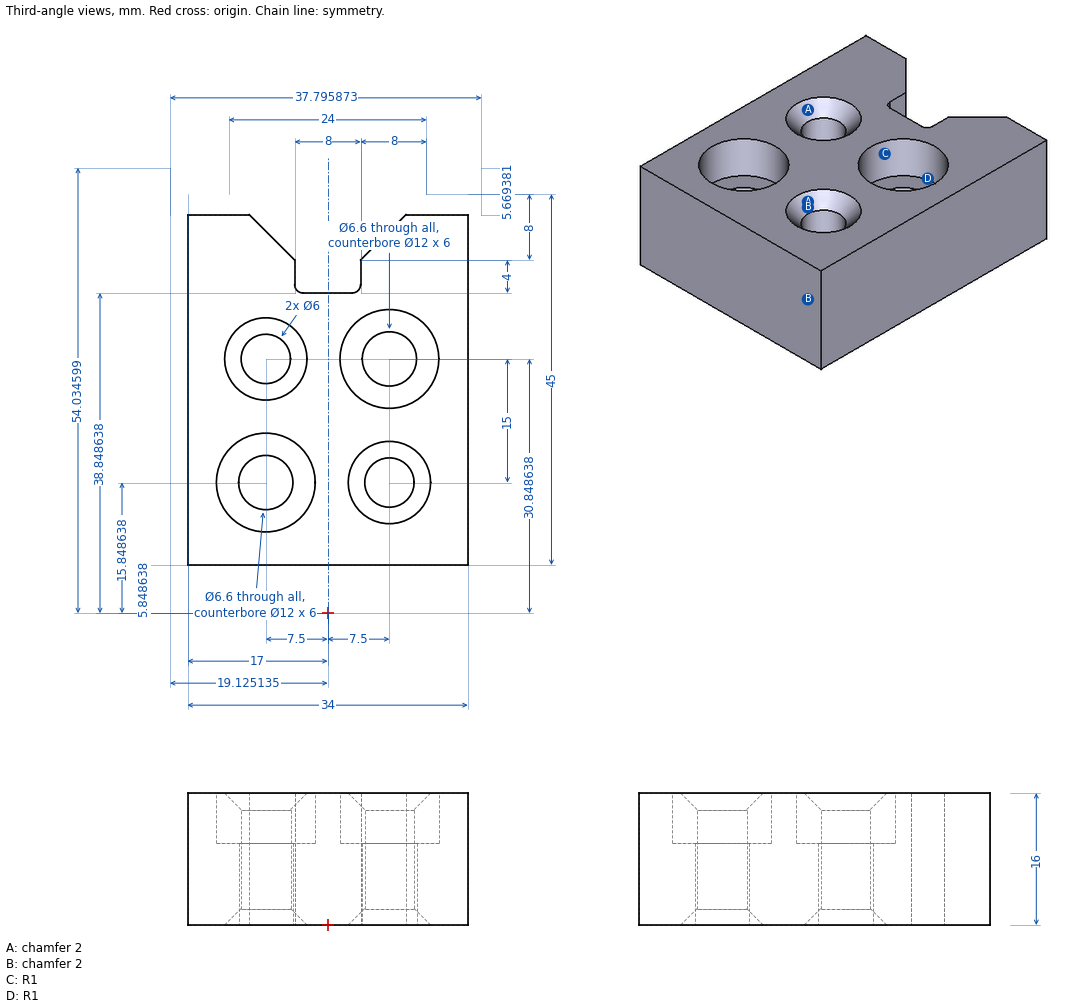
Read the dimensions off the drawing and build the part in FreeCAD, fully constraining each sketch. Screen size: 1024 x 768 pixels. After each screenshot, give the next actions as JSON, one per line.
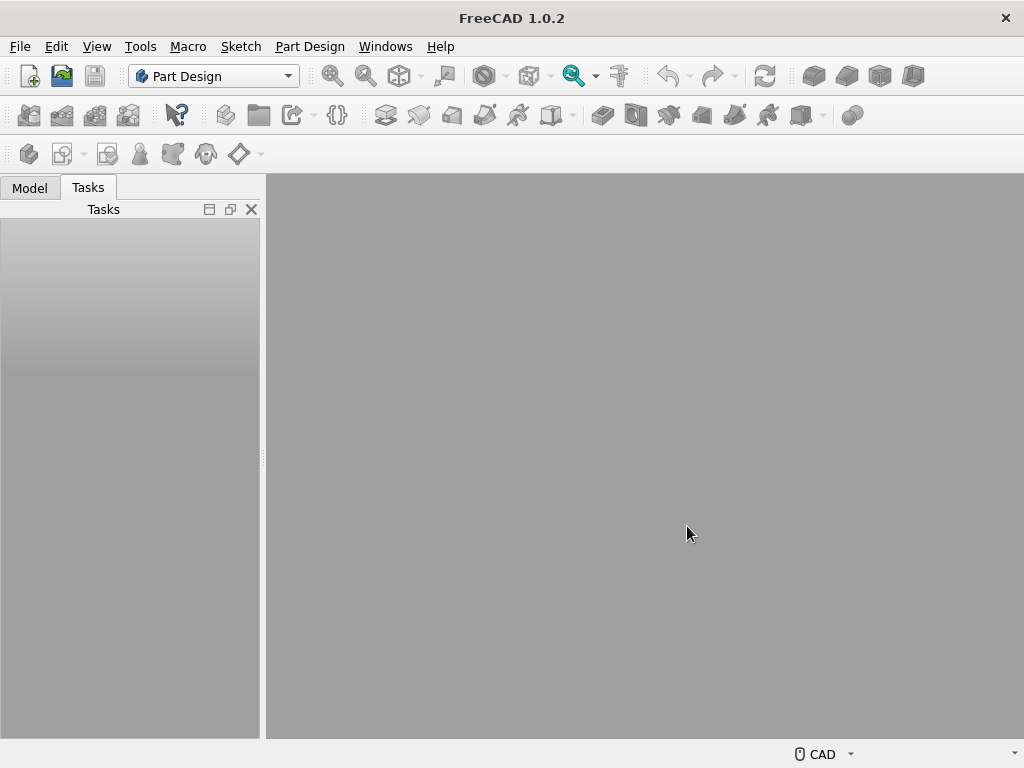
{"action": "left_click", "coordinate": [29, 76]}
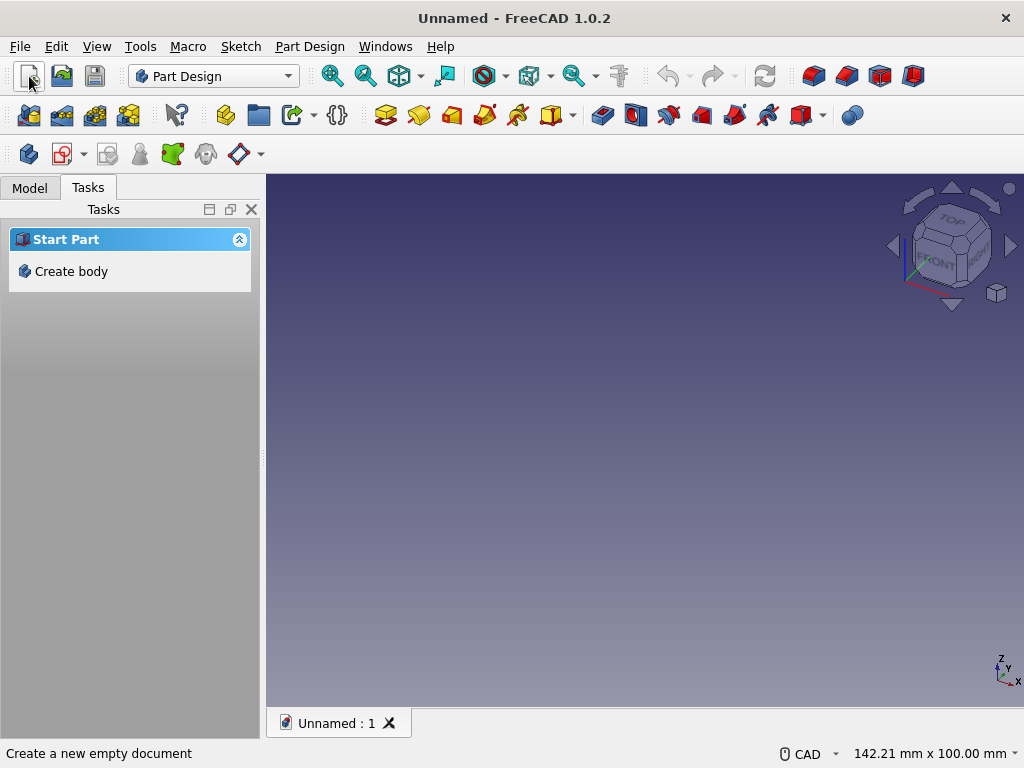
{"action": "left_click", "coordinate": [62, 154]}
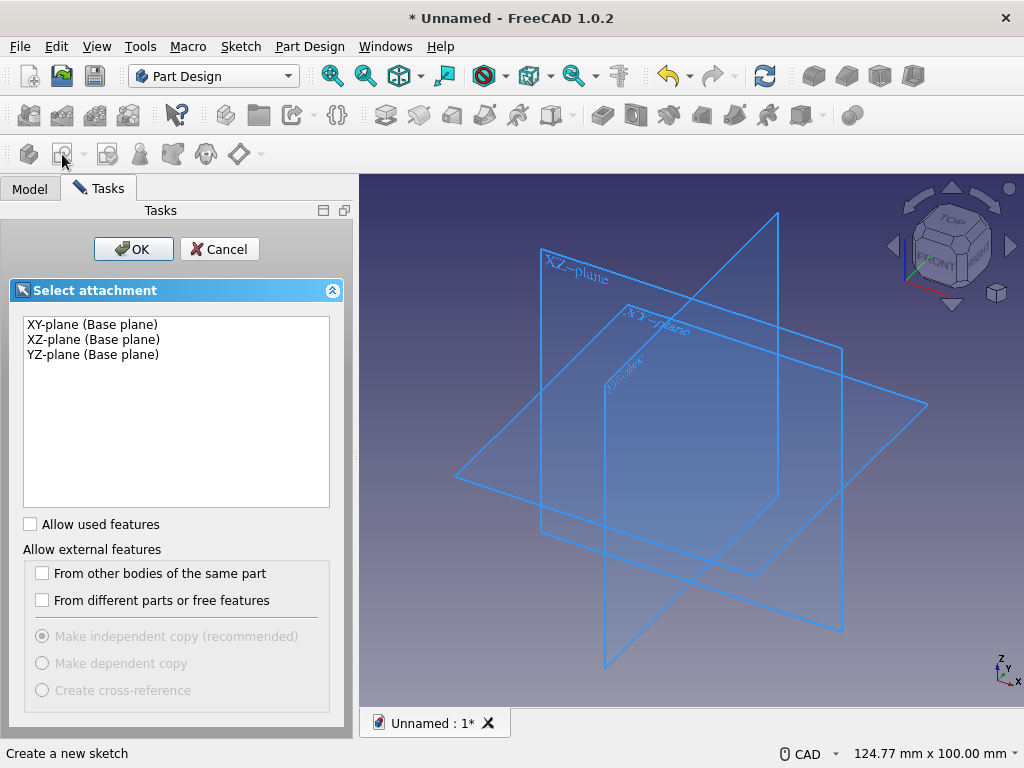
{"action": "left_click", "coordinate": [84, 324]}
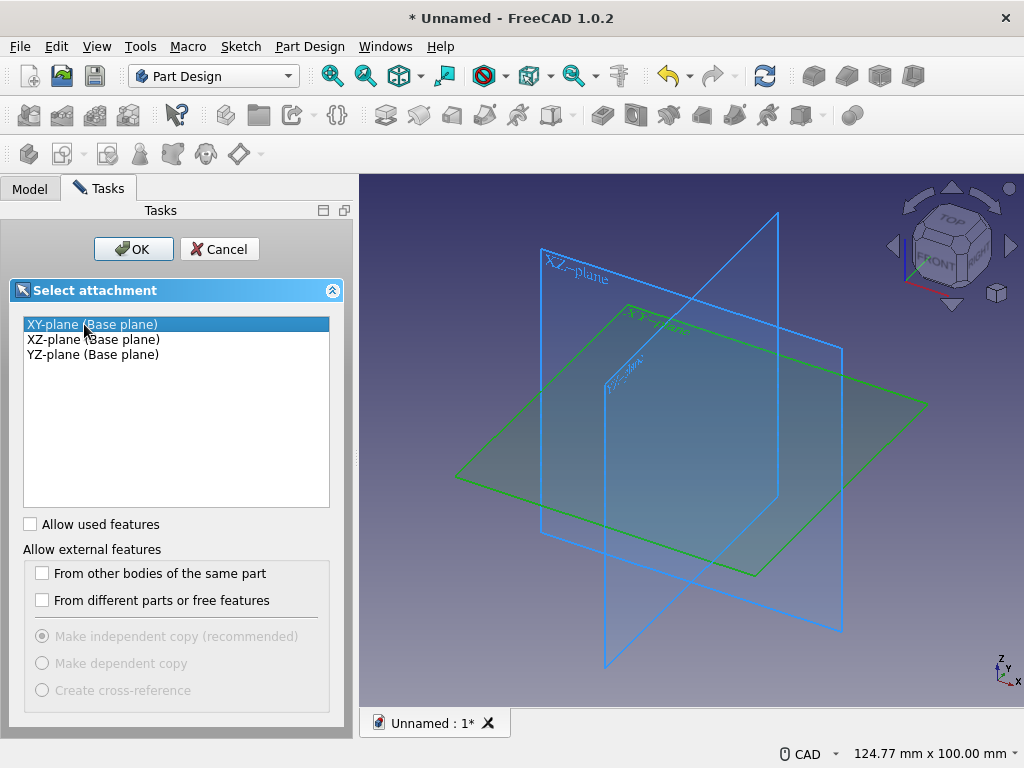
{"action": "left_click", "coordinate": [134, 249]}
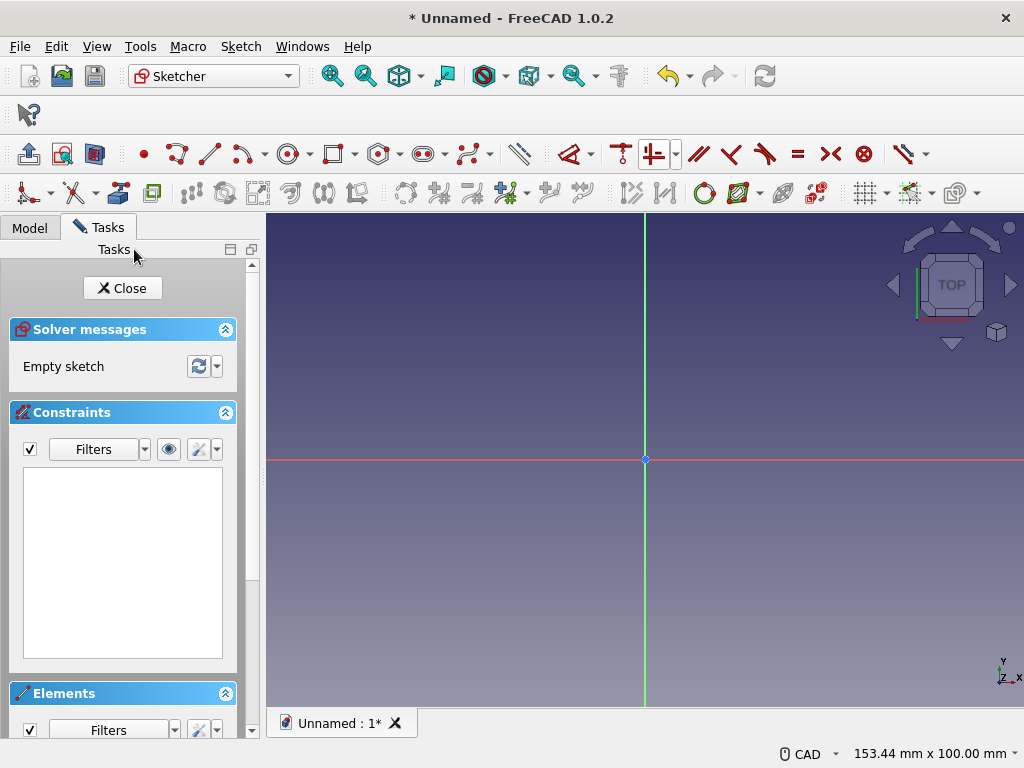
{"action": "scroll", "coordinate": [294, 679], "scroll_direction": "down", "scroll_amount": 1}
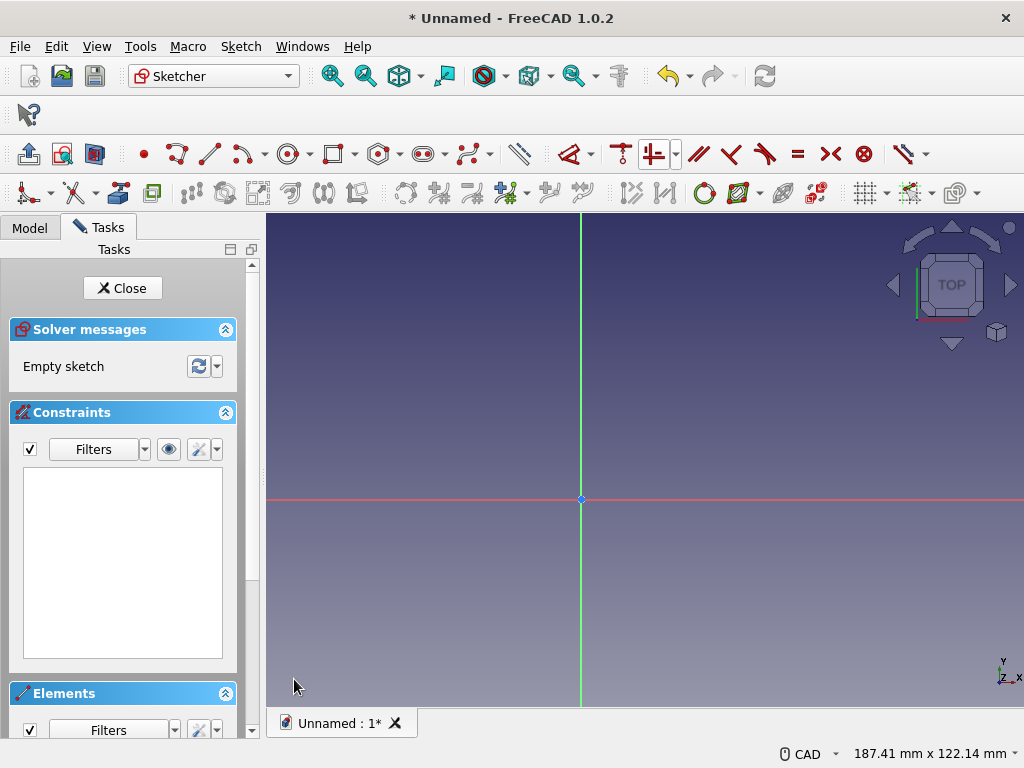
{"action": "scroll", "coordinate": [591, 269], "scroll_direction": "up", "scroll_amount": 2}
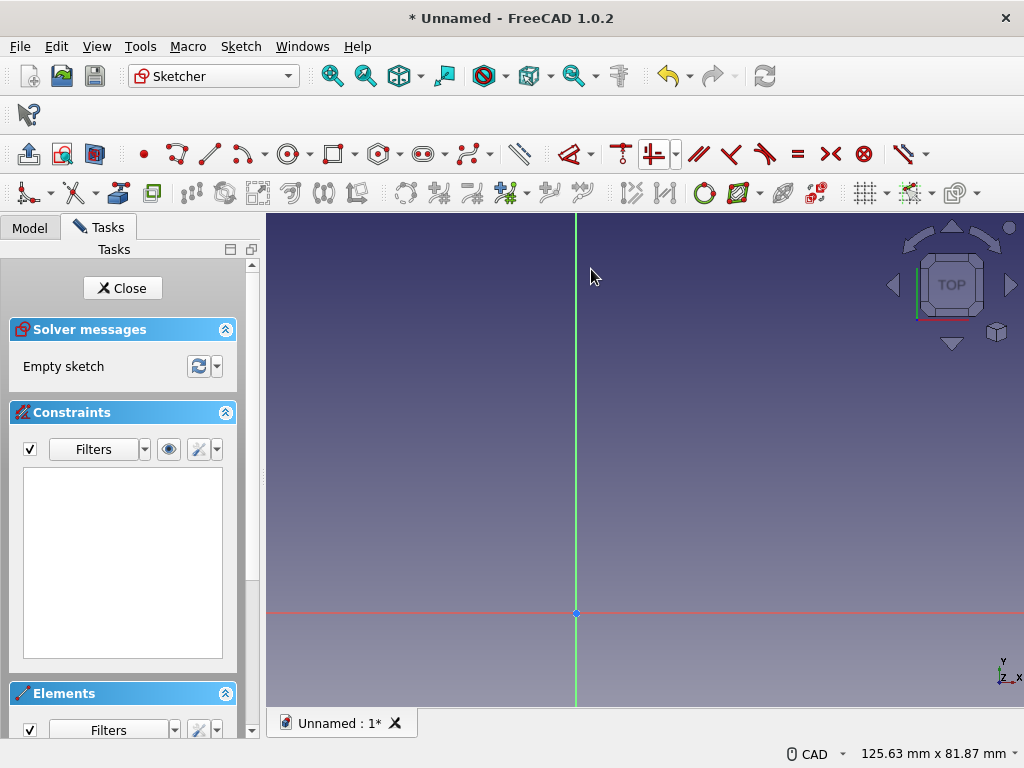
{"action": "left_click", "coordinate": [332, 154]}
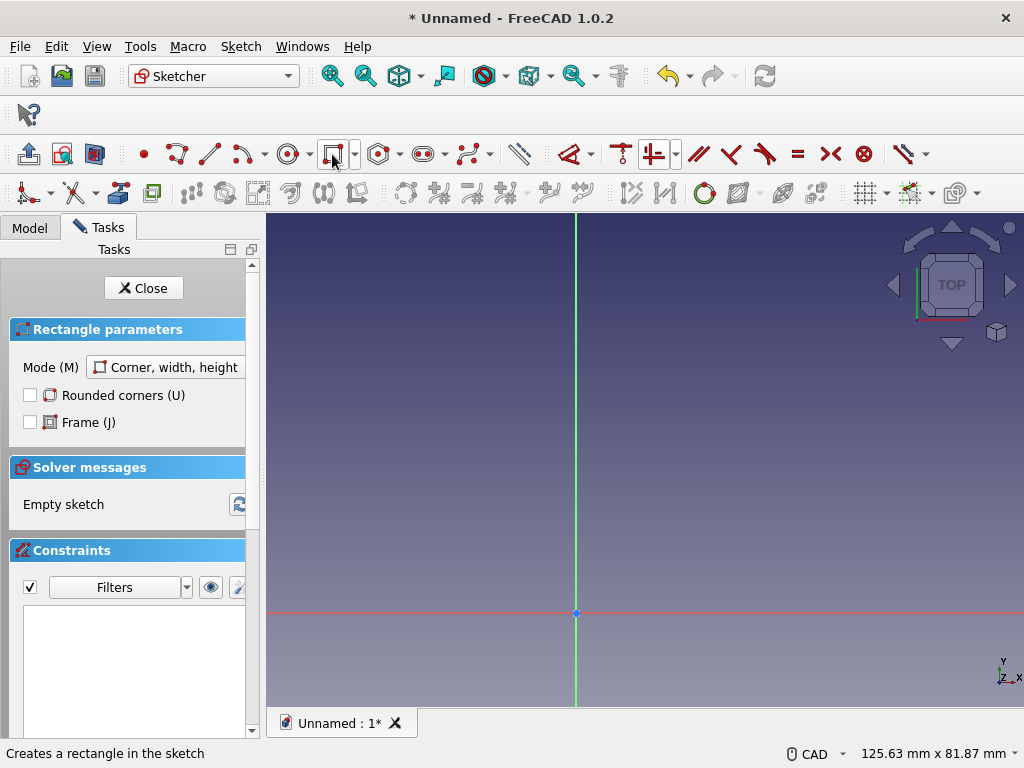
{"action": "left_click", "coordinate": [474, 307]}
{"action": "mouse_move", "coordinate": [679, 578]}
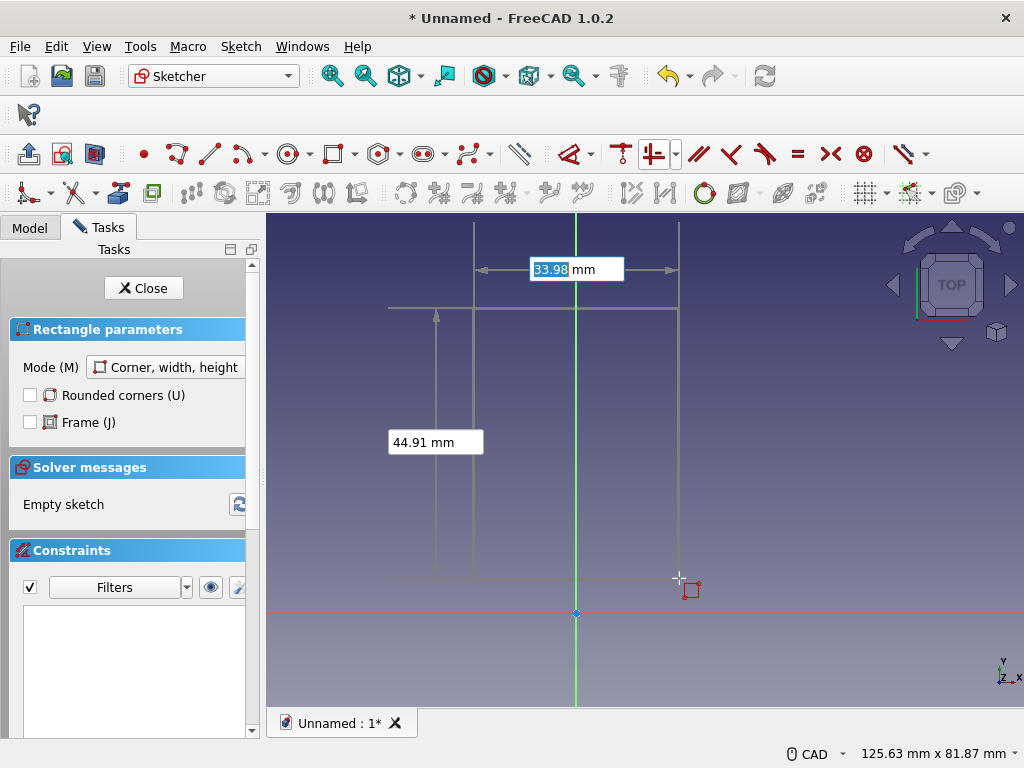
{"action": "type", "text": "34"}
{"action": "key", "text": "Tab"}
{"action": "type", "text": "45"}
{"action": "key", "text": "Return"}
{"action": "key", "text": "Escape"}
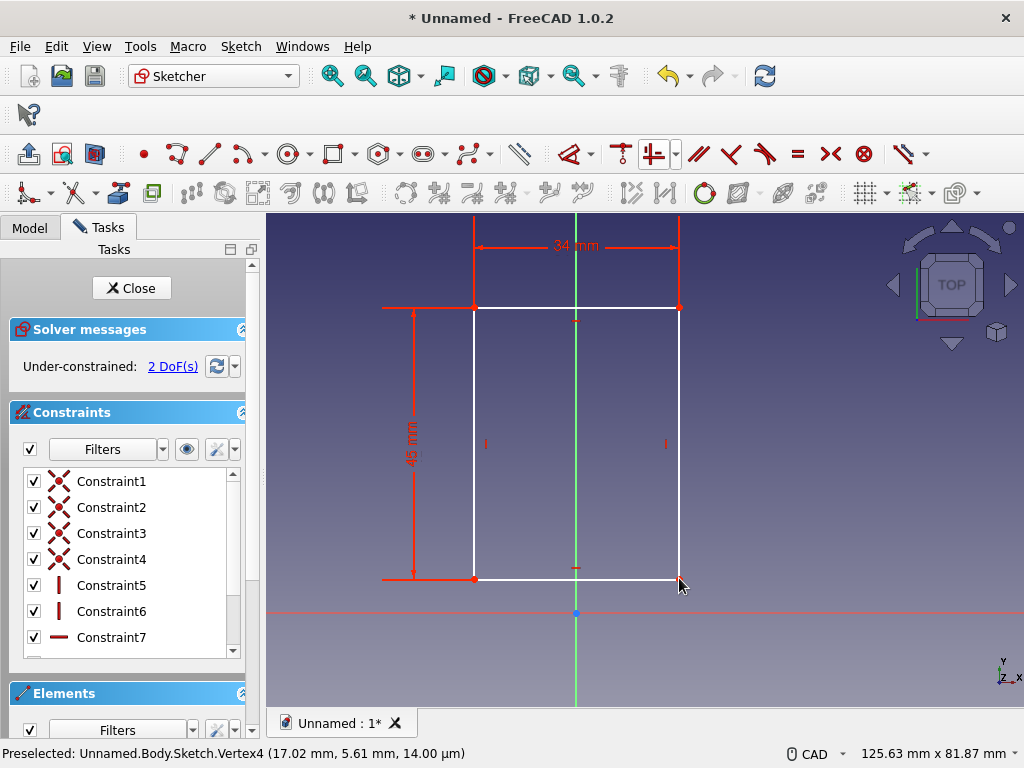
{"action": "left_click", "coordinate": [568, 154]}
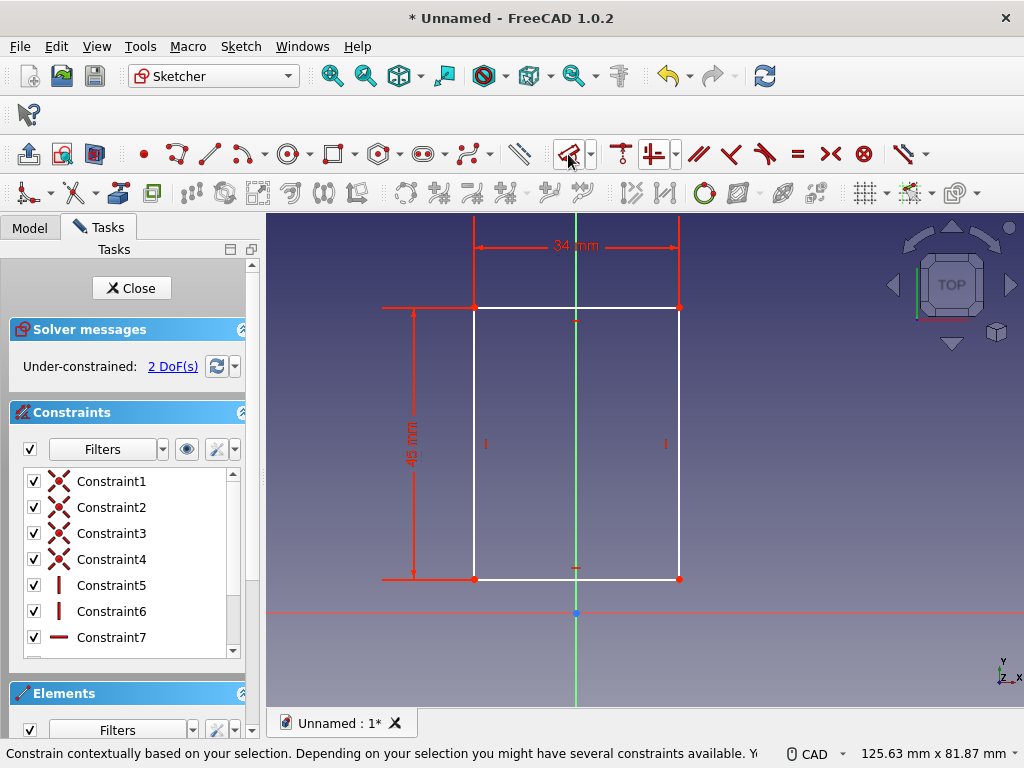
{"action": "left_click", "coordinate": [474, 308]}
{"action": "left_click", "coordinate": [525, 647]}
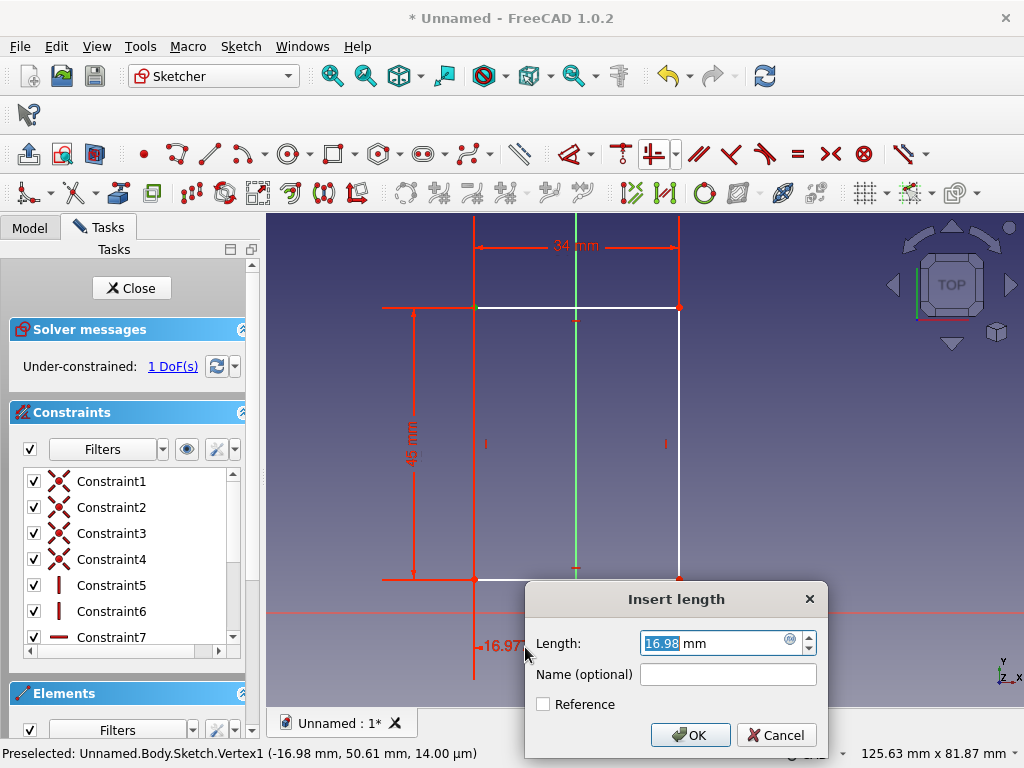
{"action": "type", "text": "17"}
{"action": "key", "text": "Return"}